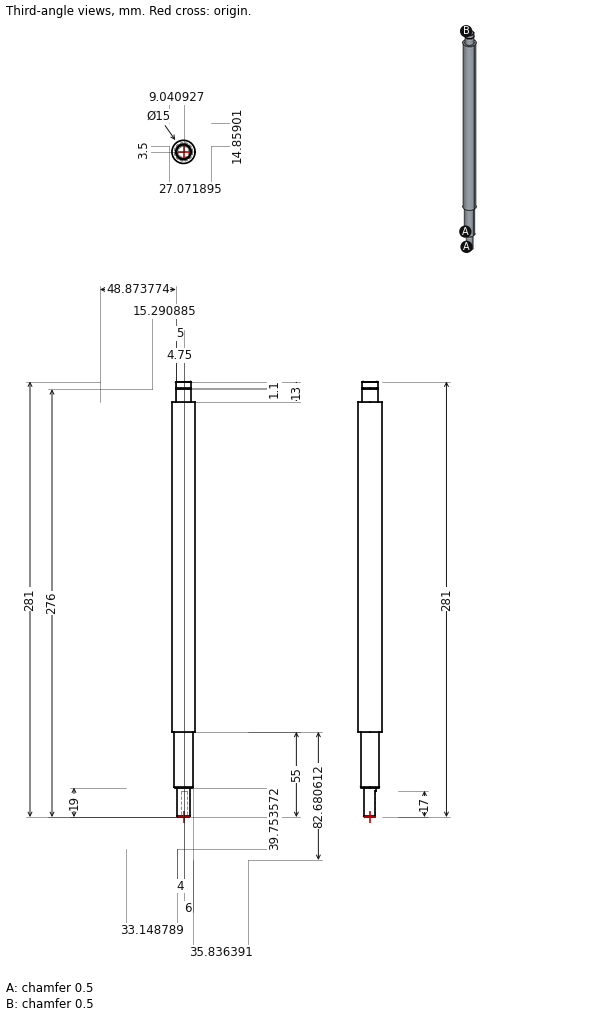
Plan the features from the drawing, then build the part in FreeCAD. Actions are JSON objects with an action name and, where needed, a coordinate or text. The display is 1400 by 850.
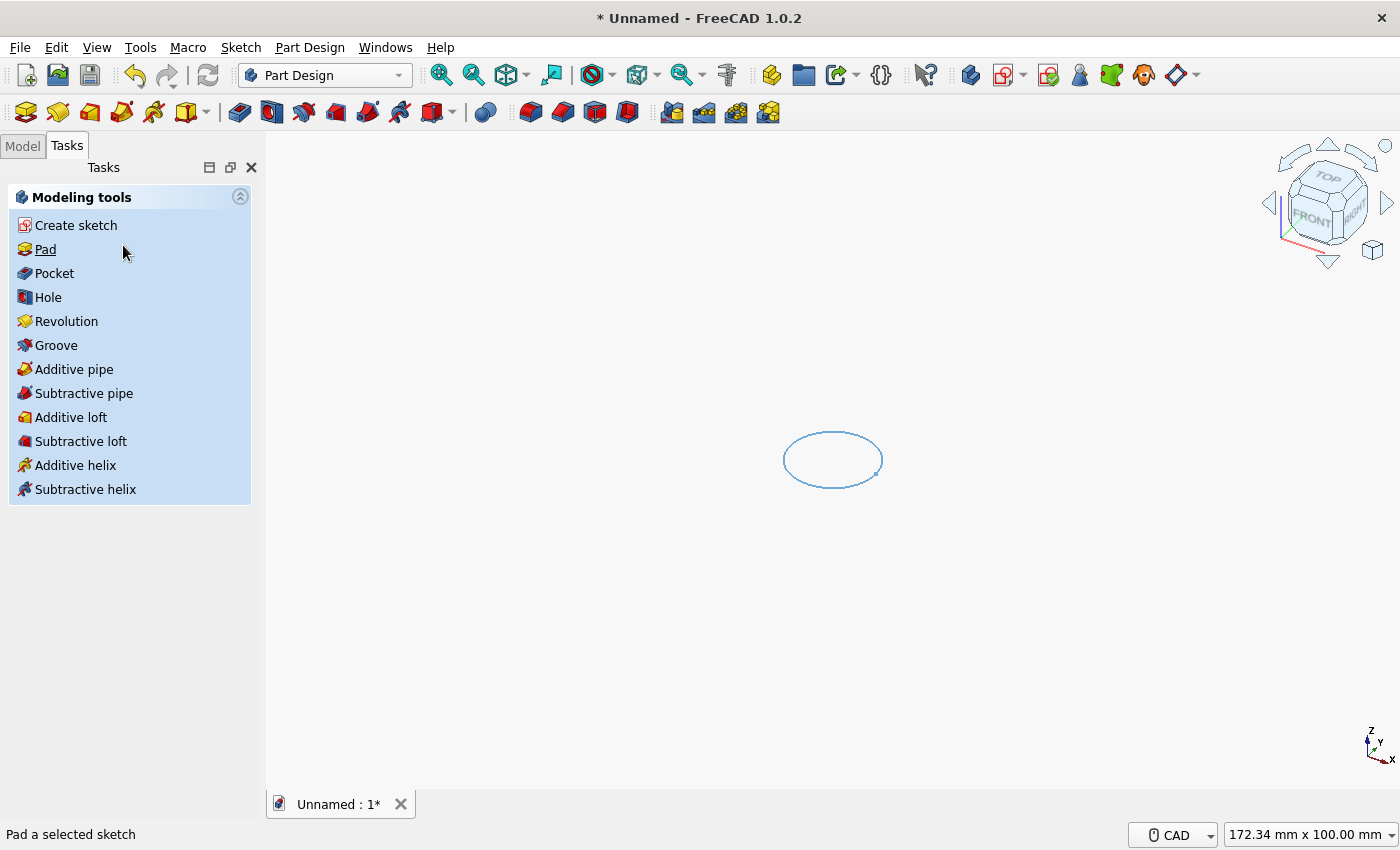
{"action": "left_click", "coordinate": [26, 112]}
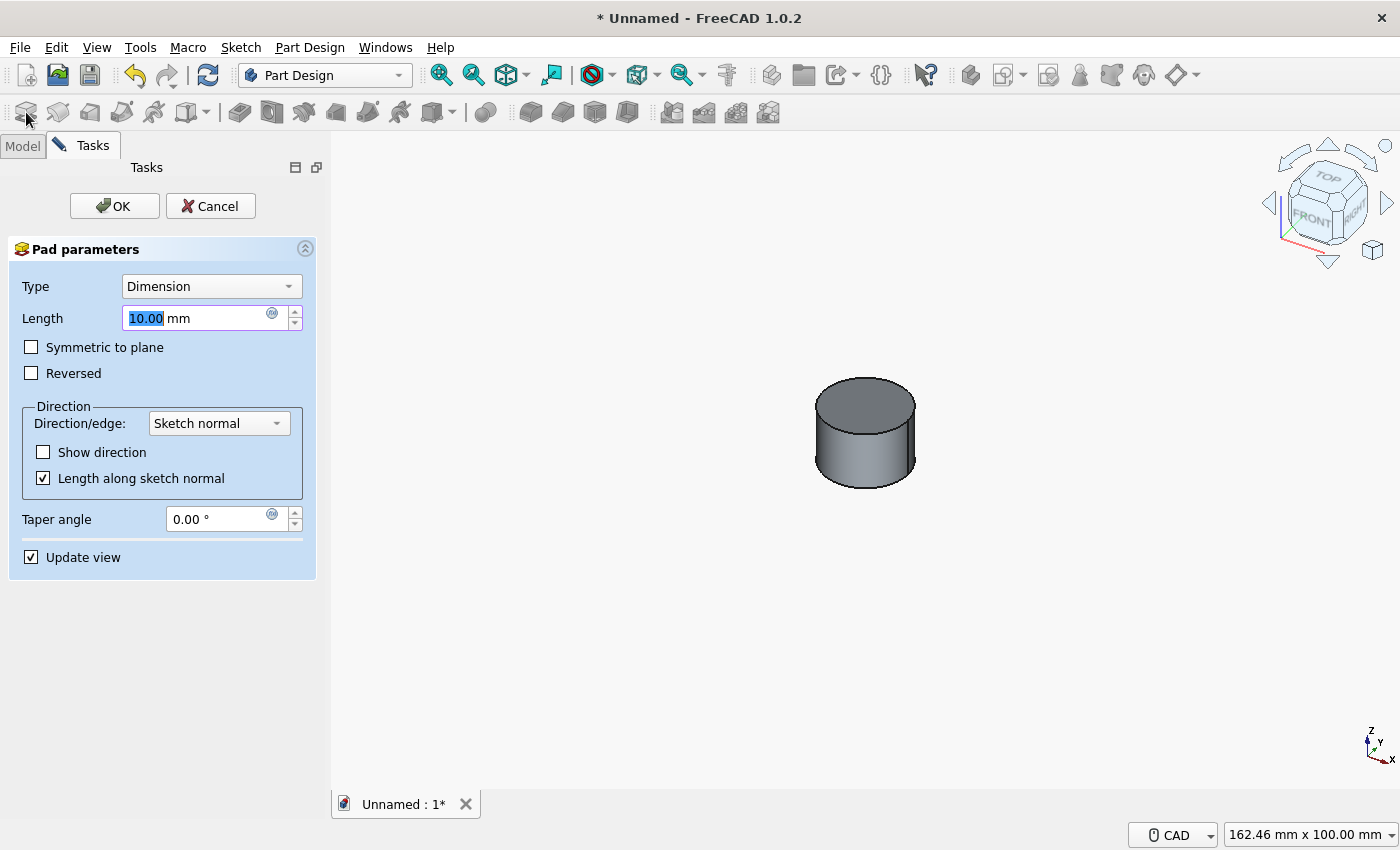
{"action": "type", "text": "281"}
{"action": "key", "text": "Tab"}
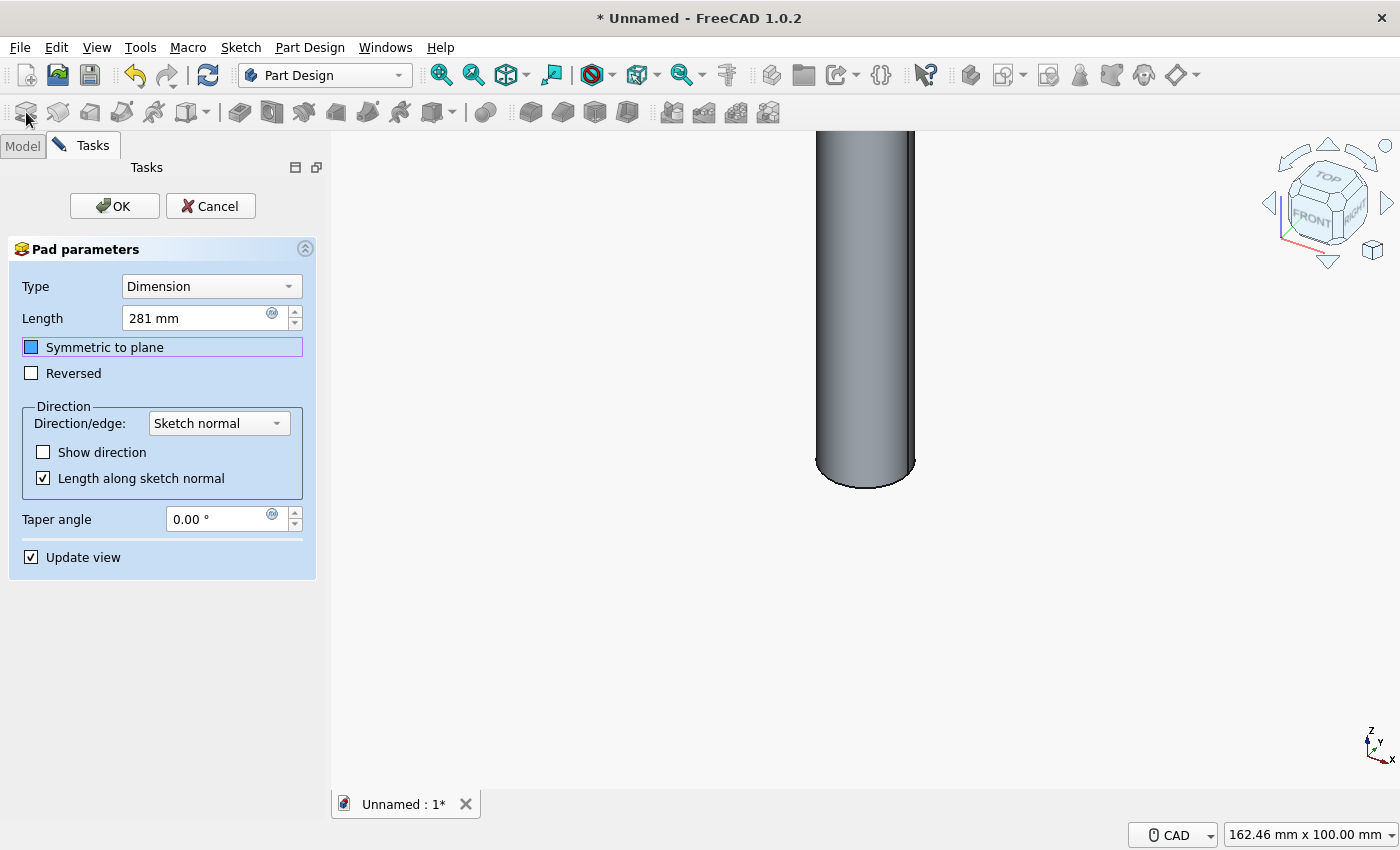
{"action": "left_click", "coordinate": [115, 206]}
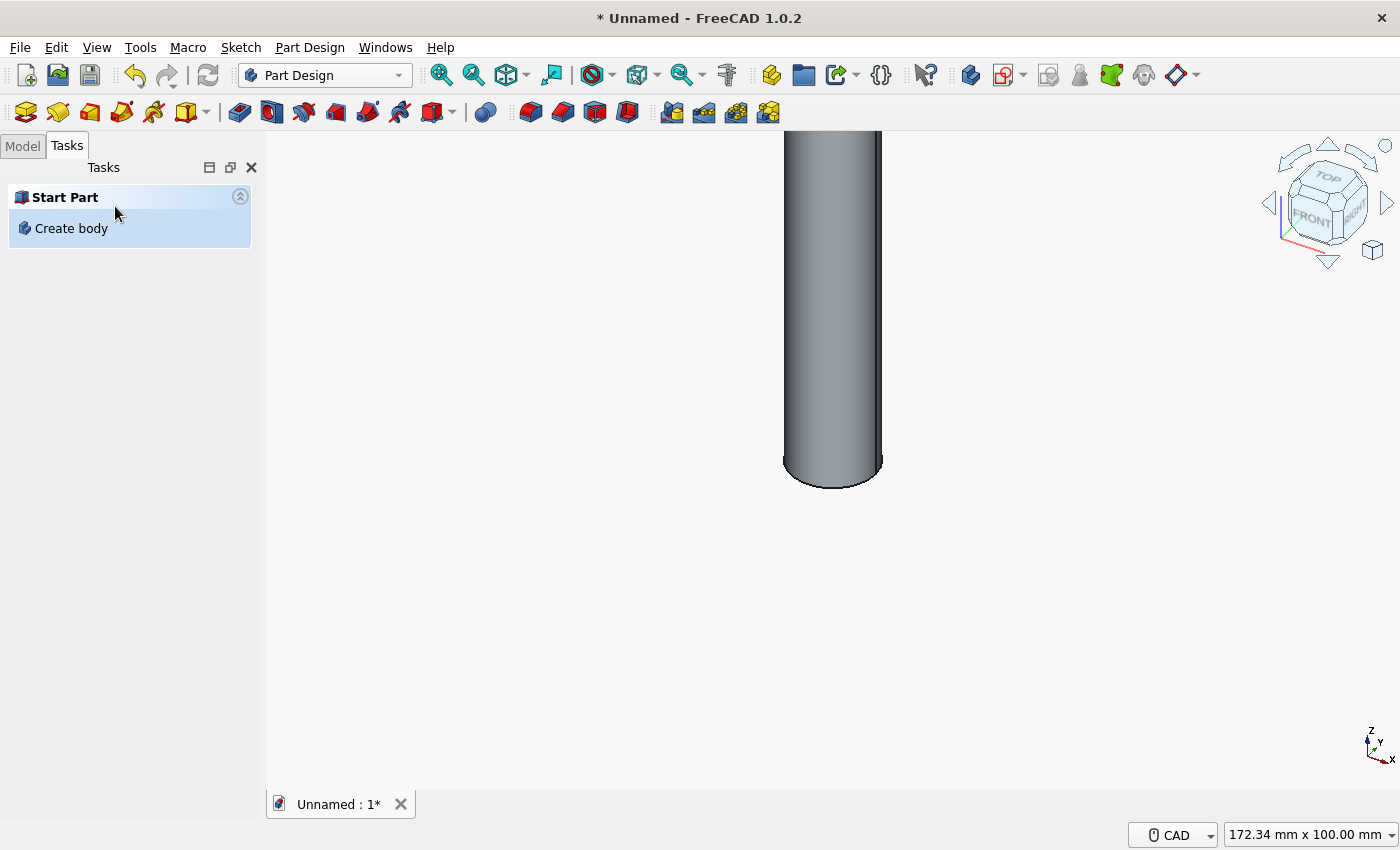
{"action": "left_click", "coordinate": [442, 76]}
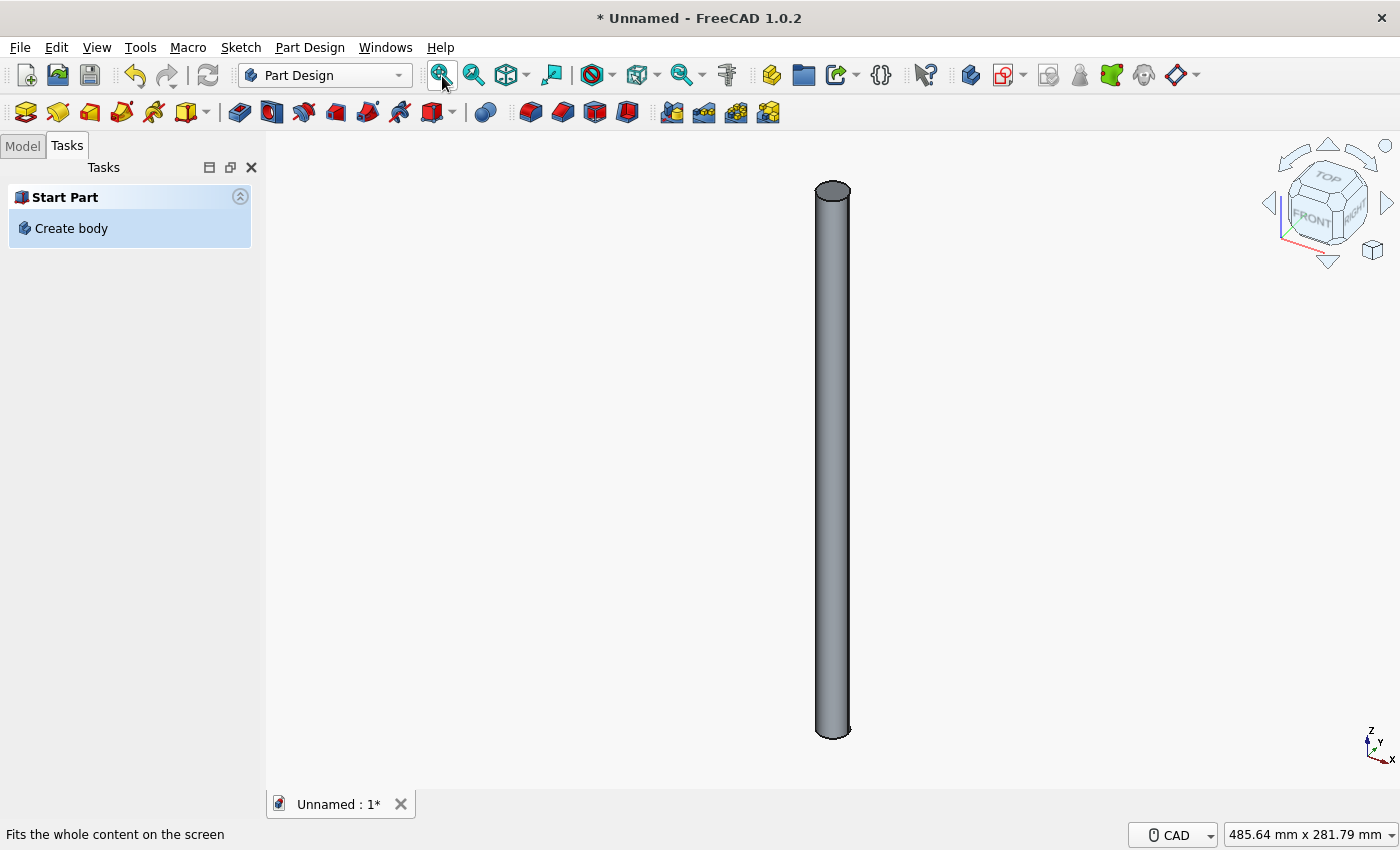
{"action": "left_click", "coordinate": [1004, 76]}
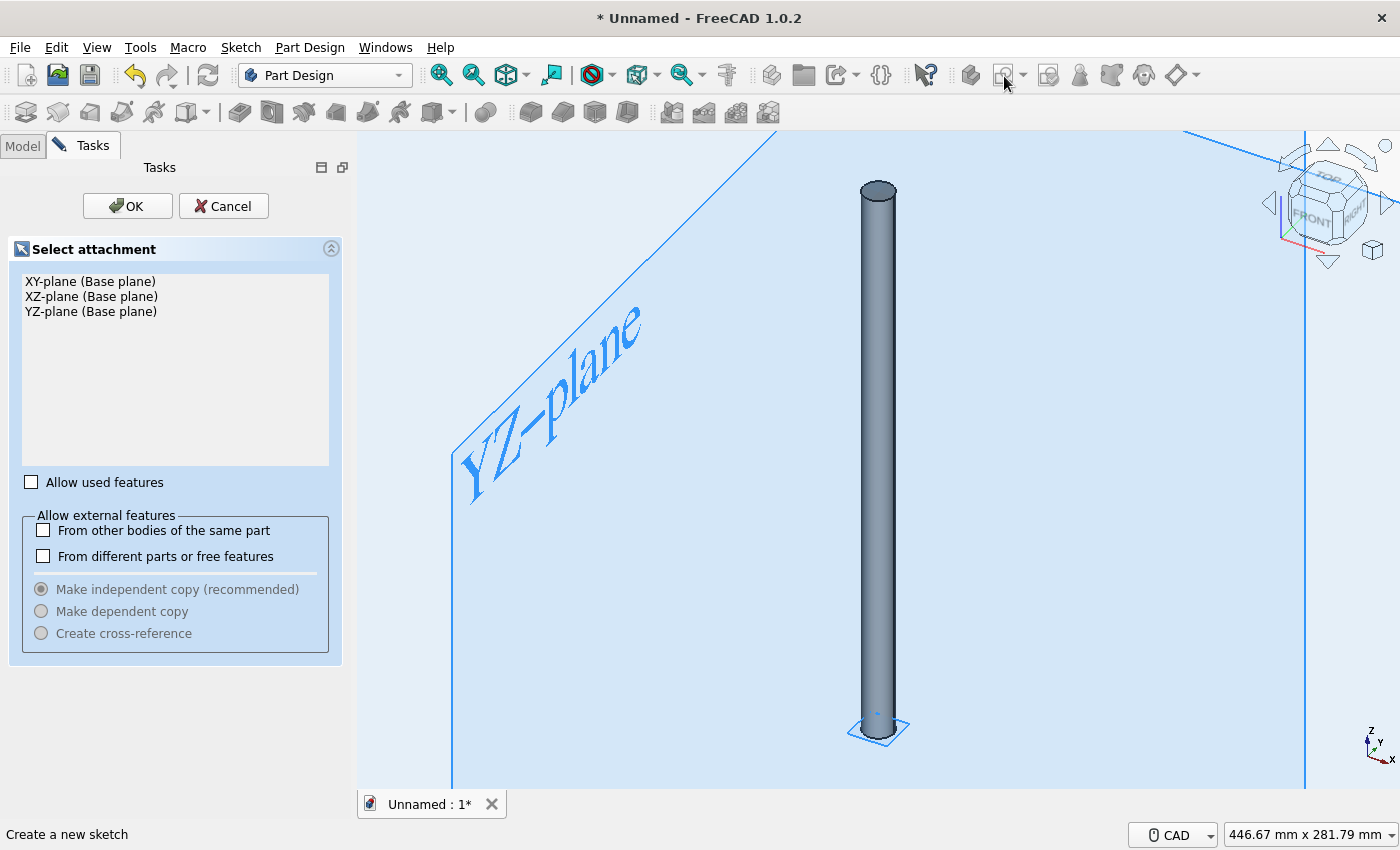
{"action": "left_click", "coordinate": [82, 296]}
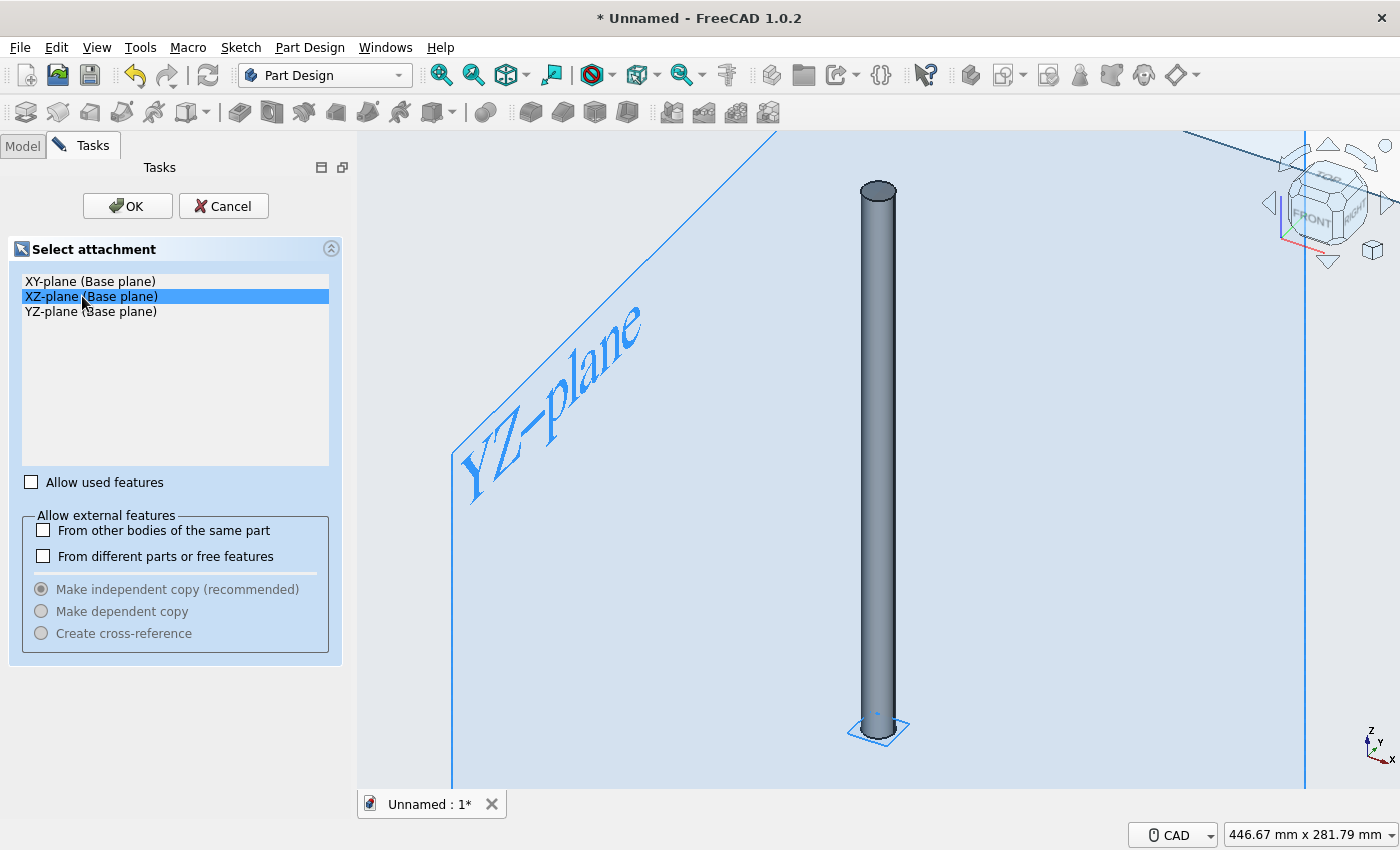
{"action": "left_click", "coordinate": [128, 206]}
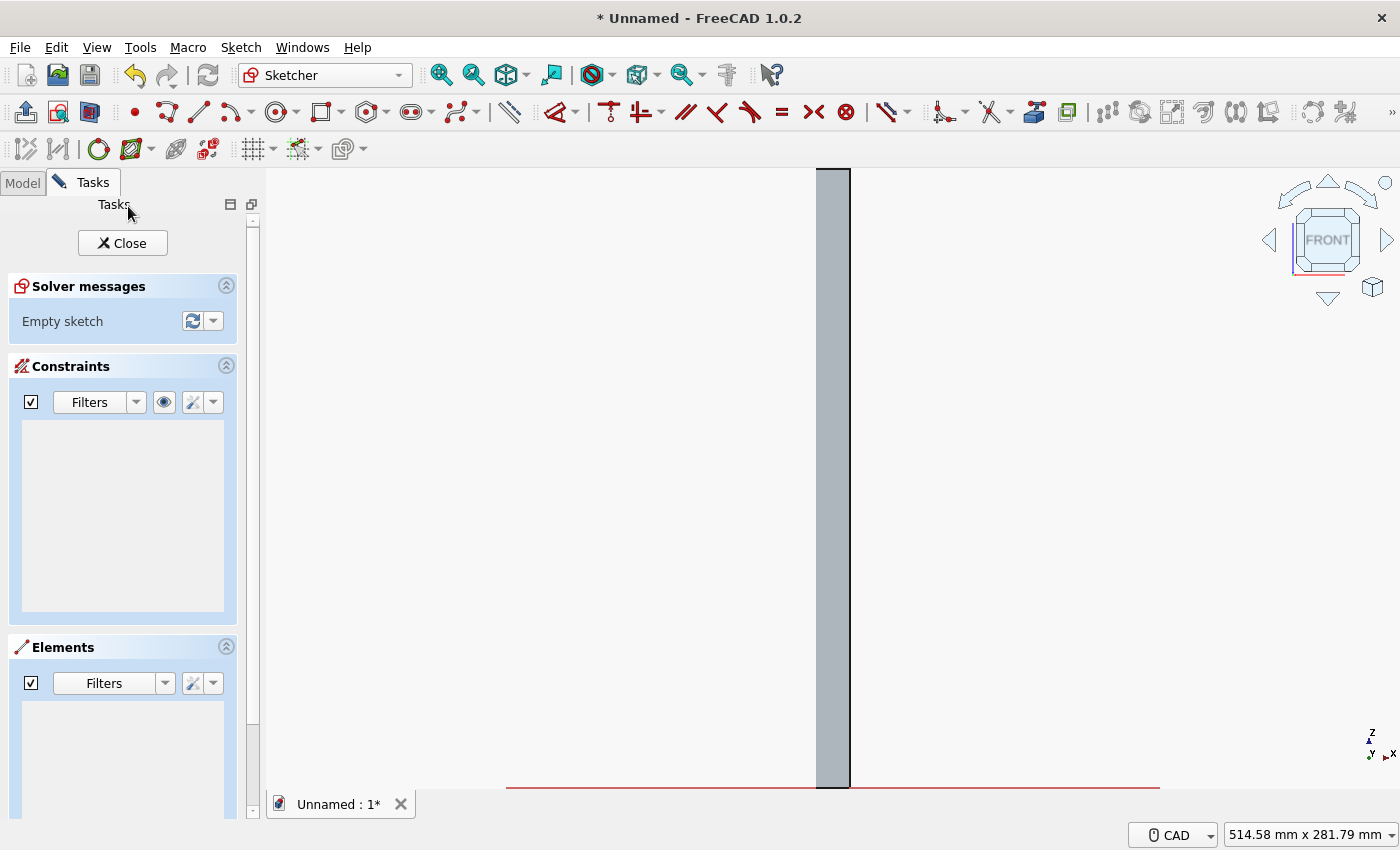
{"action": "left_click", "coordinate": [90, 112]}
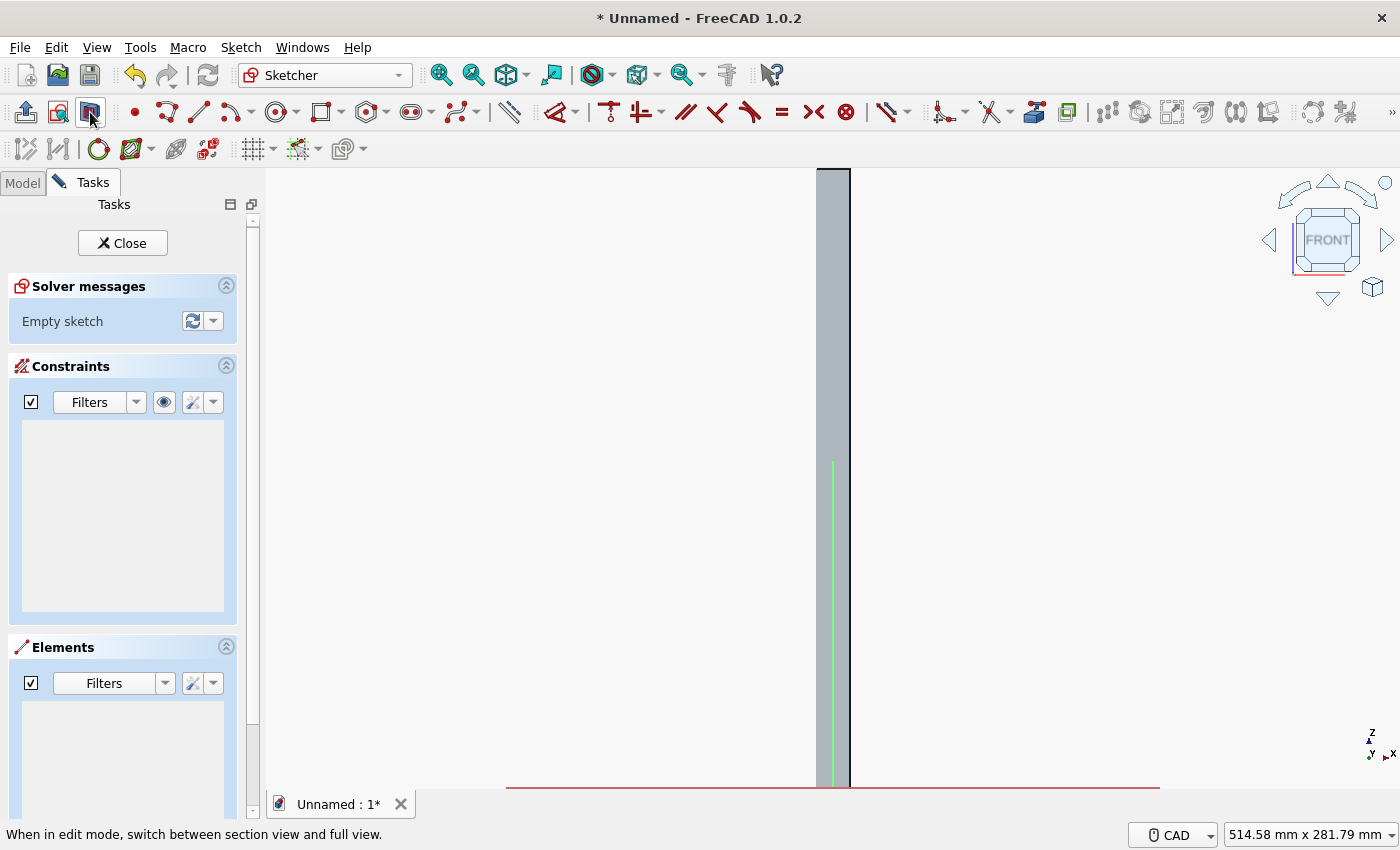
{"action": "scroll", "coordinate": [764, 478], "scroll_direction": "down", "scroll_amount": 5}